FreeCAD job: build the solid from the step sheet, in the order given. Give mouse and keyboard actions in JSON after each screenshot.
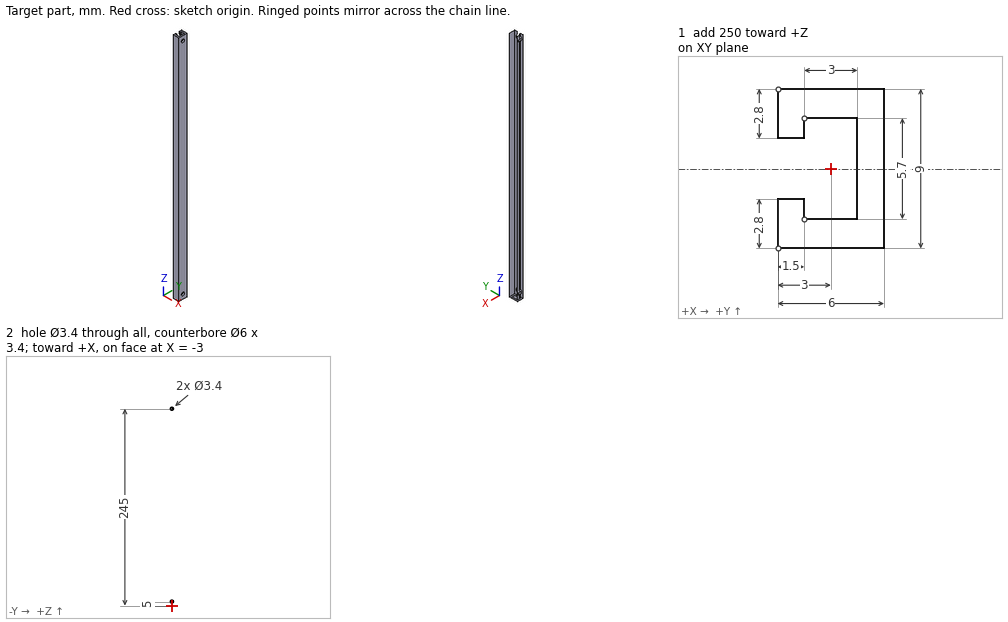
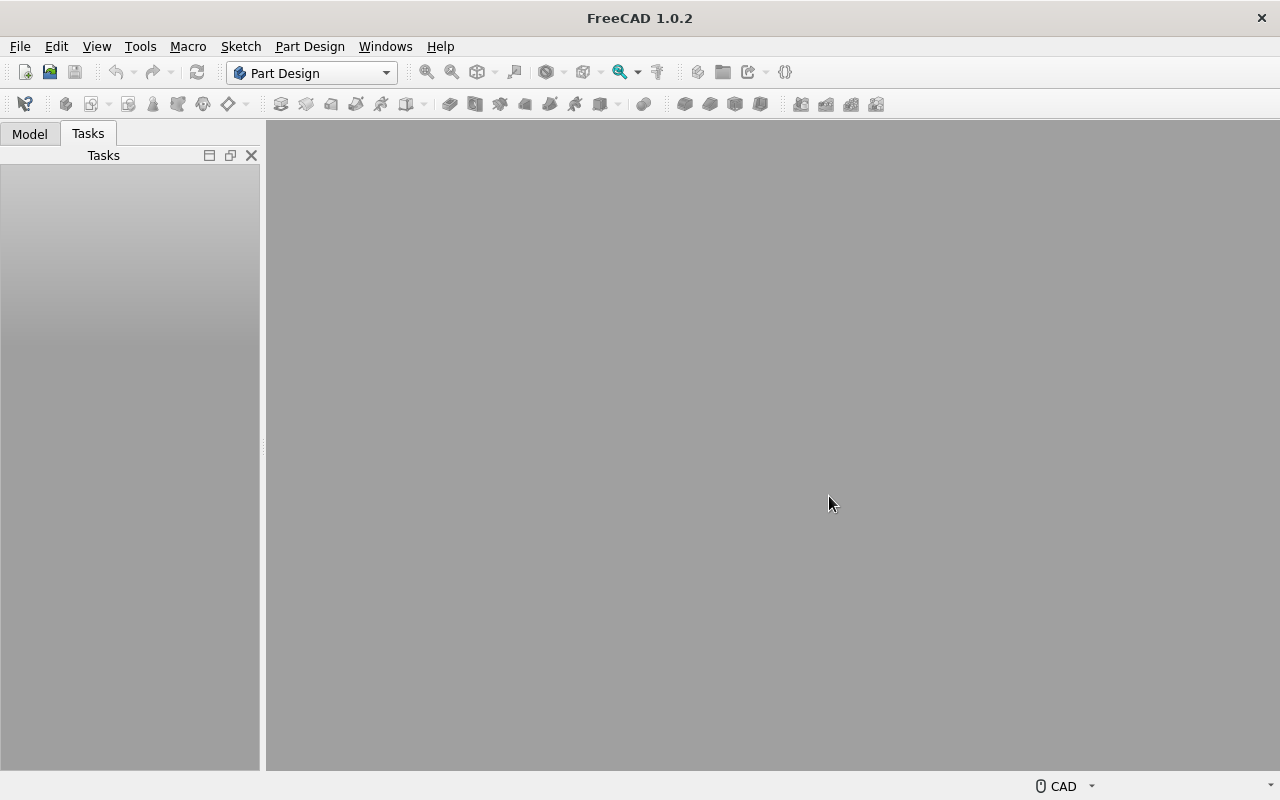
{"action": "left_click", "coordinate": [25, 72]}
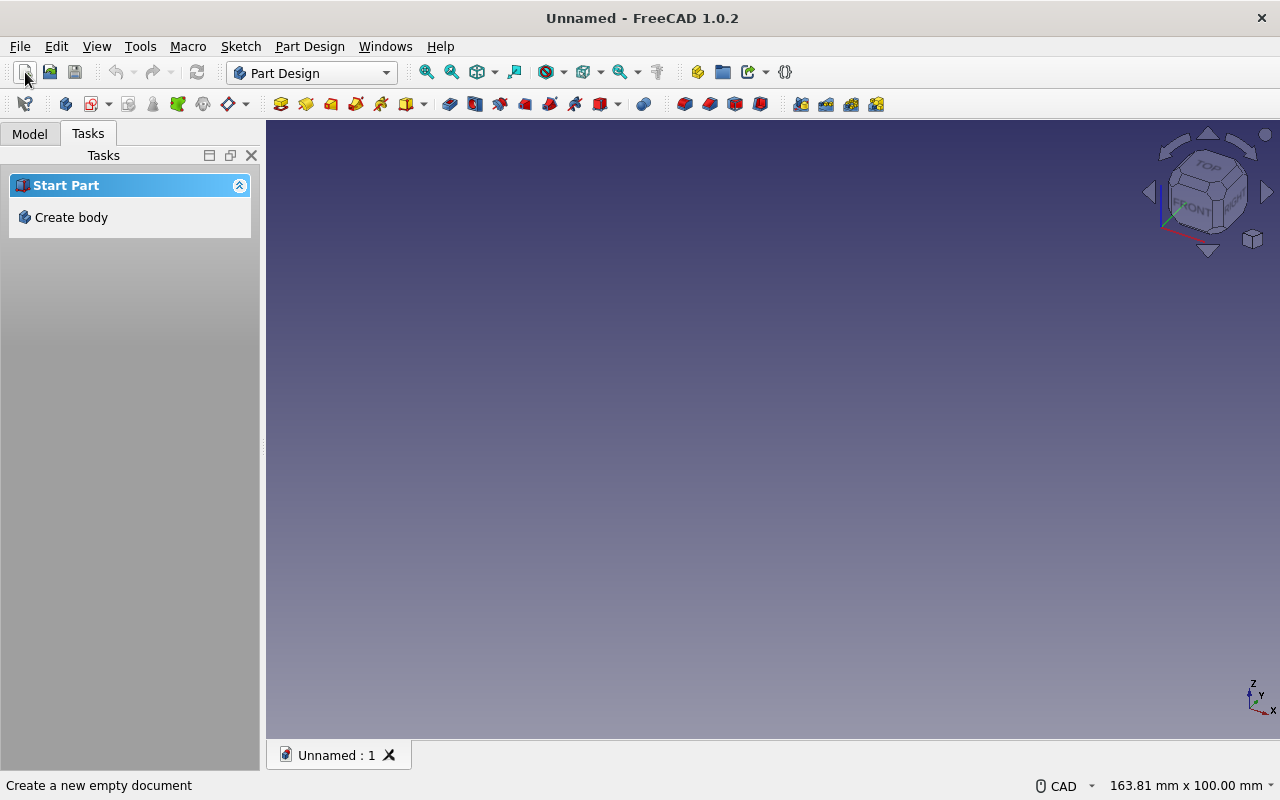
{"action": "left_click", "coordinate": [90, 104]}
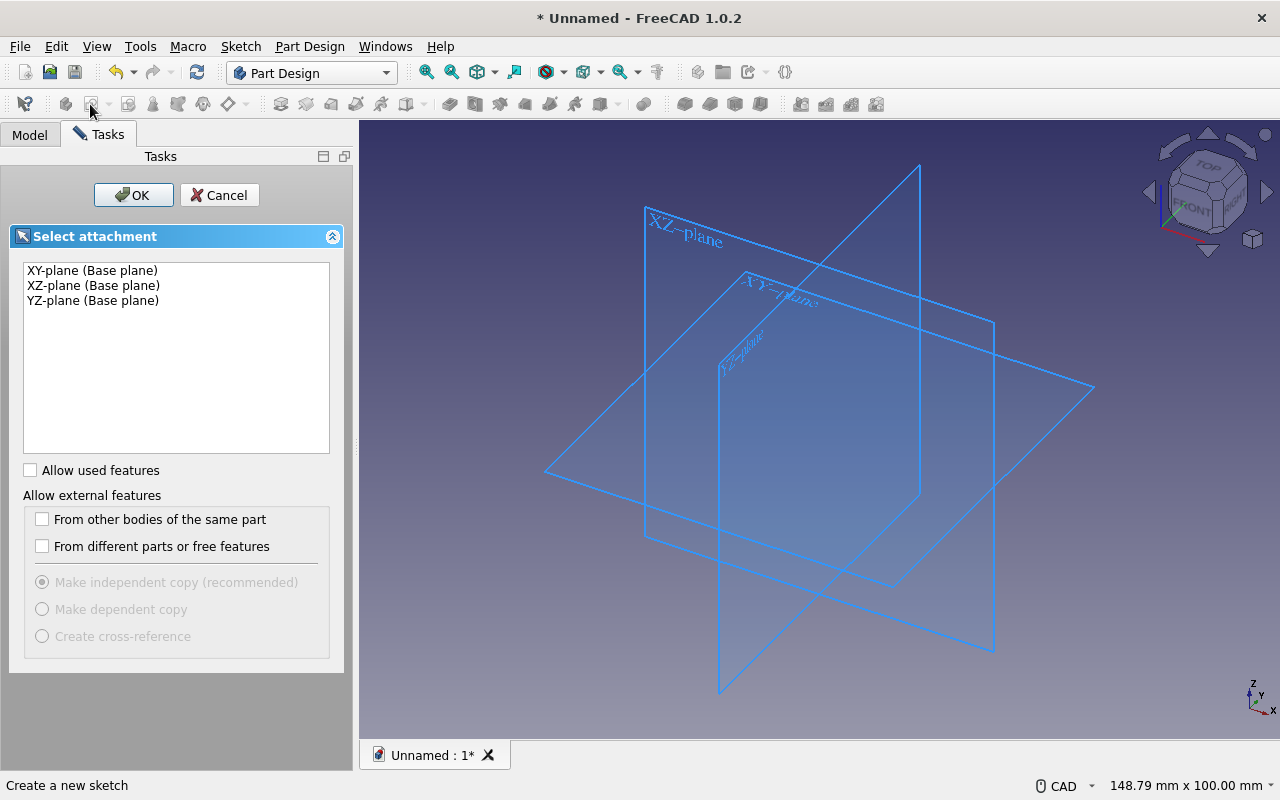
{"action": "left_click", "coordinate": [84, 270]}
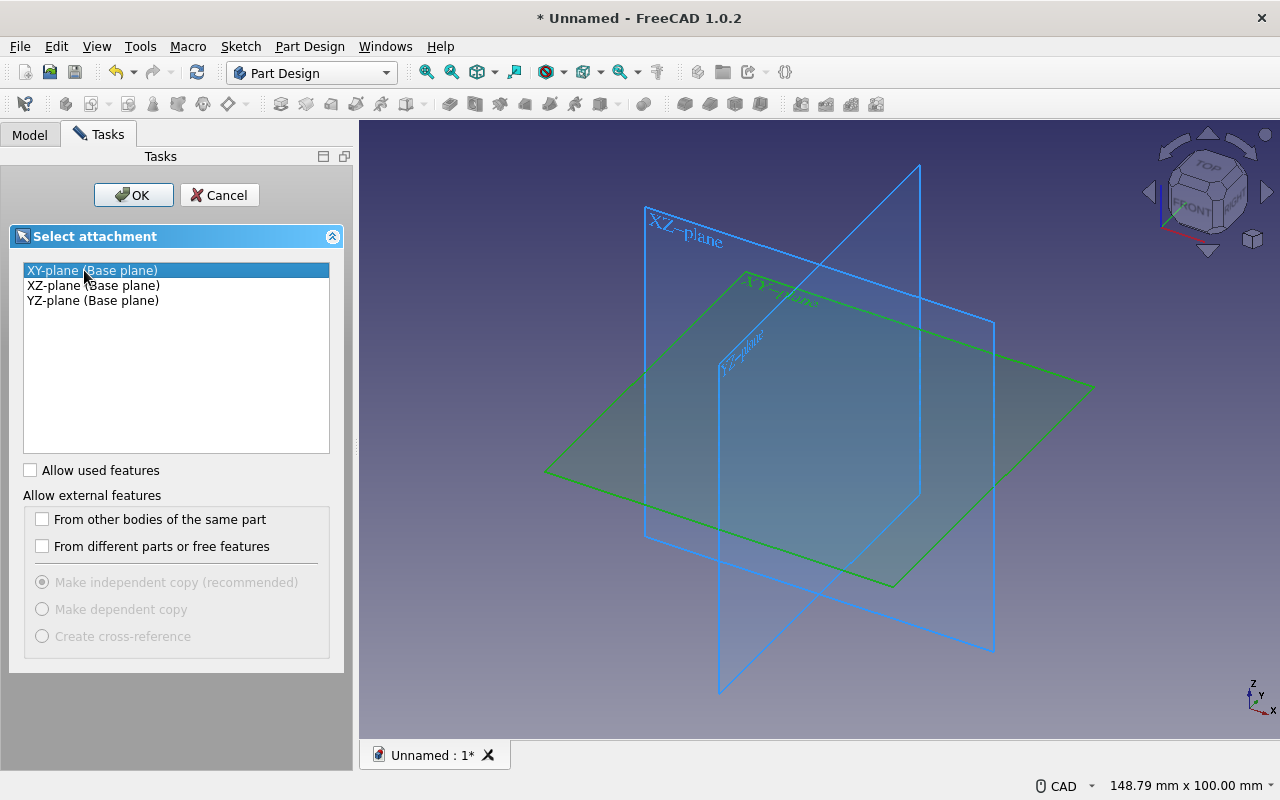
{"action": "left_click", "coordinate": [134, 195]}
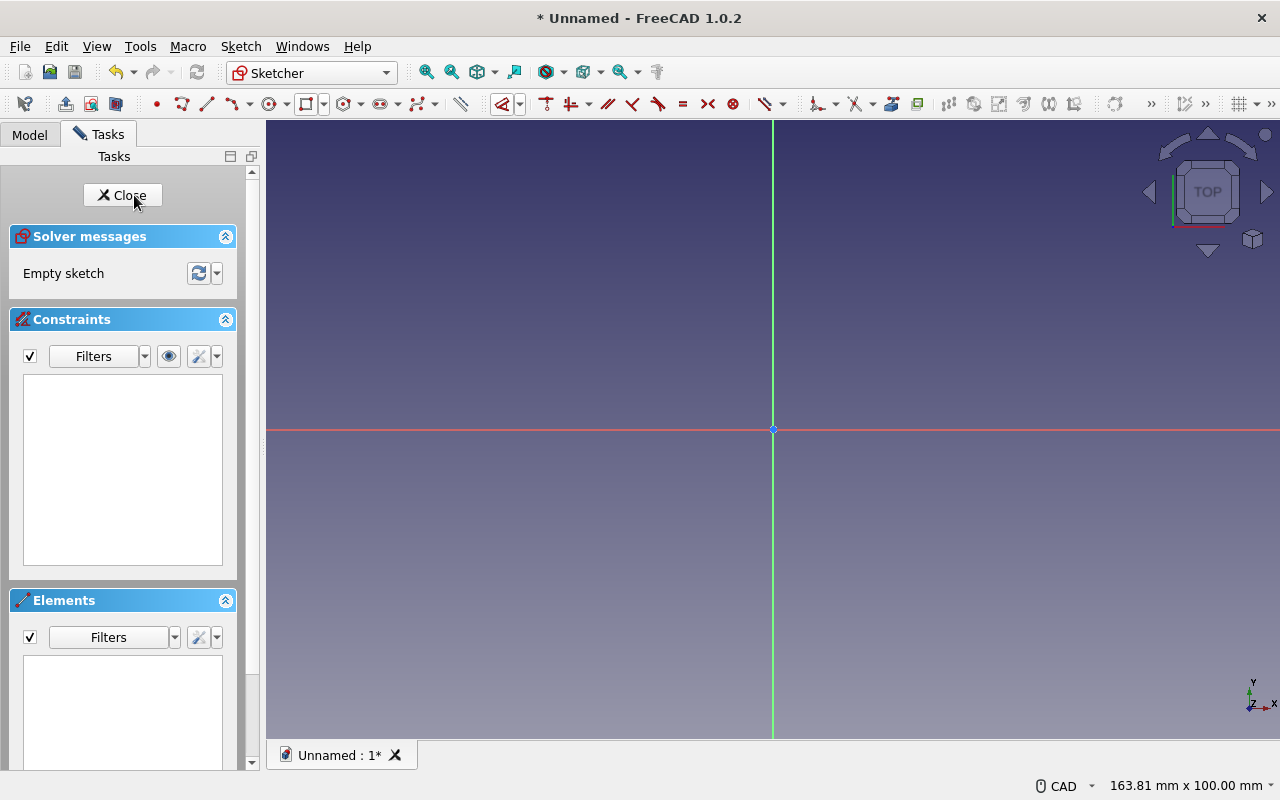
{"action": "scroll", "coordinate": [784, 430], "scroll_direction": "up", "scroll_amount": 10}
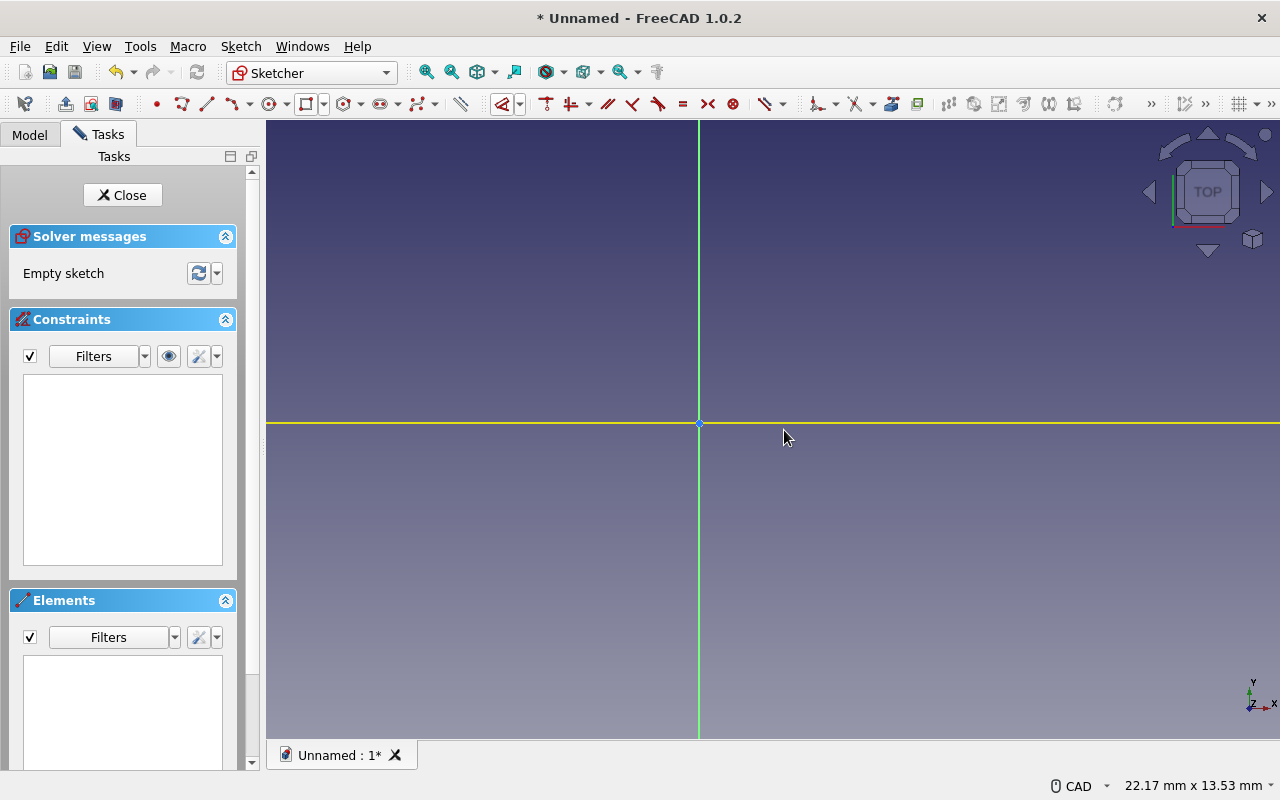
{"action": "key", "text": "g m"}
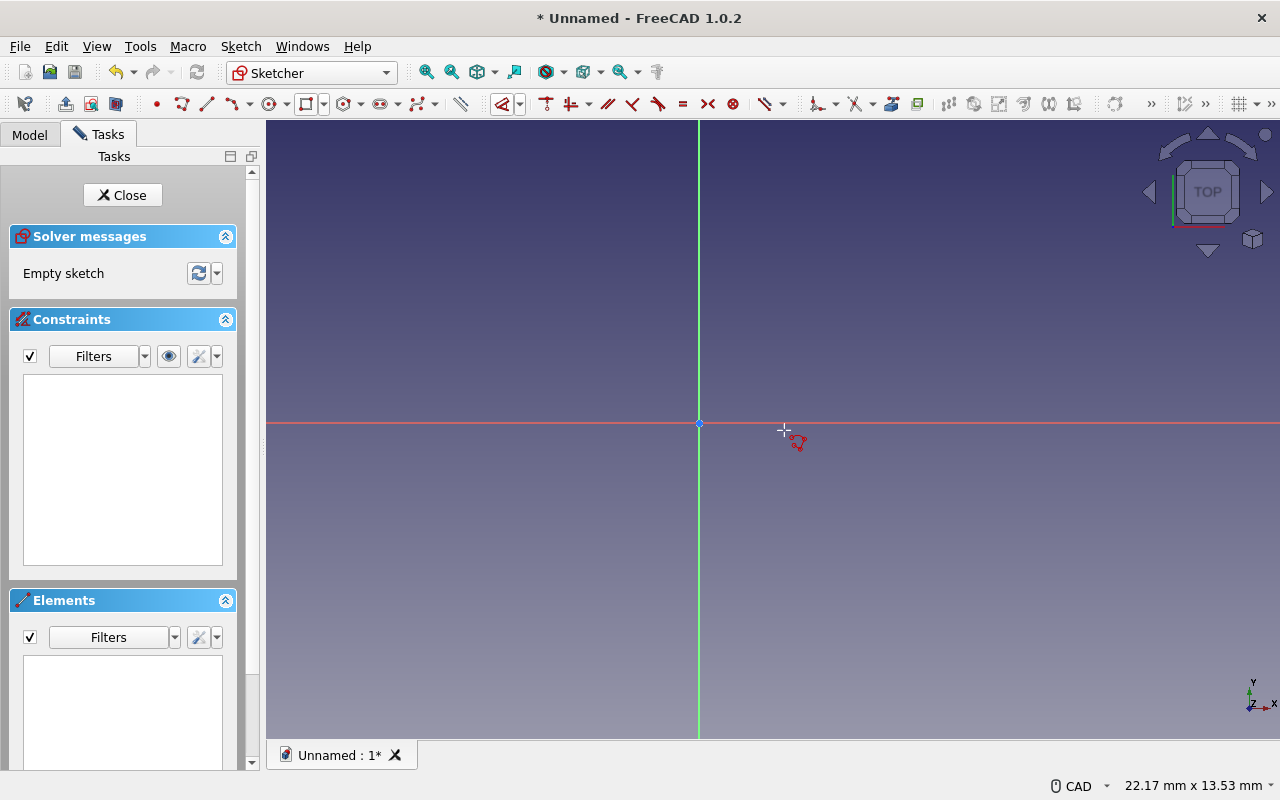
{"action": "left_click", "coordinate": [631, 345]}
{"action": "left_click", "coordinate": [631, 293]}
{"action": "left_click", "coordinate": [768, 293]}
{"action": "left_click", "coordinate": [768, 553]}
{"action": "left_click", "coordinate": [631, 553]}
{"action": "left_click", "coordinate": [631, 501]}
{"action": "left_click", "coordinate": [562, 501]}
{"action": "left_click", "coordinate": [562, 629]}
{"action": "left_click", "coordinate": [837, 629]}
{"action": "left_click", "coordinate": [837, 217]}
{"action": "left_click", "coordinate": [562, 217]}
{"action": "left_click", "coordinate": [562, 345]}
{"action": "left_click", "coordinate": [631, 346]}
{"action": "key", "text": "Escape"}
{"action": "key", "text": "Escape"}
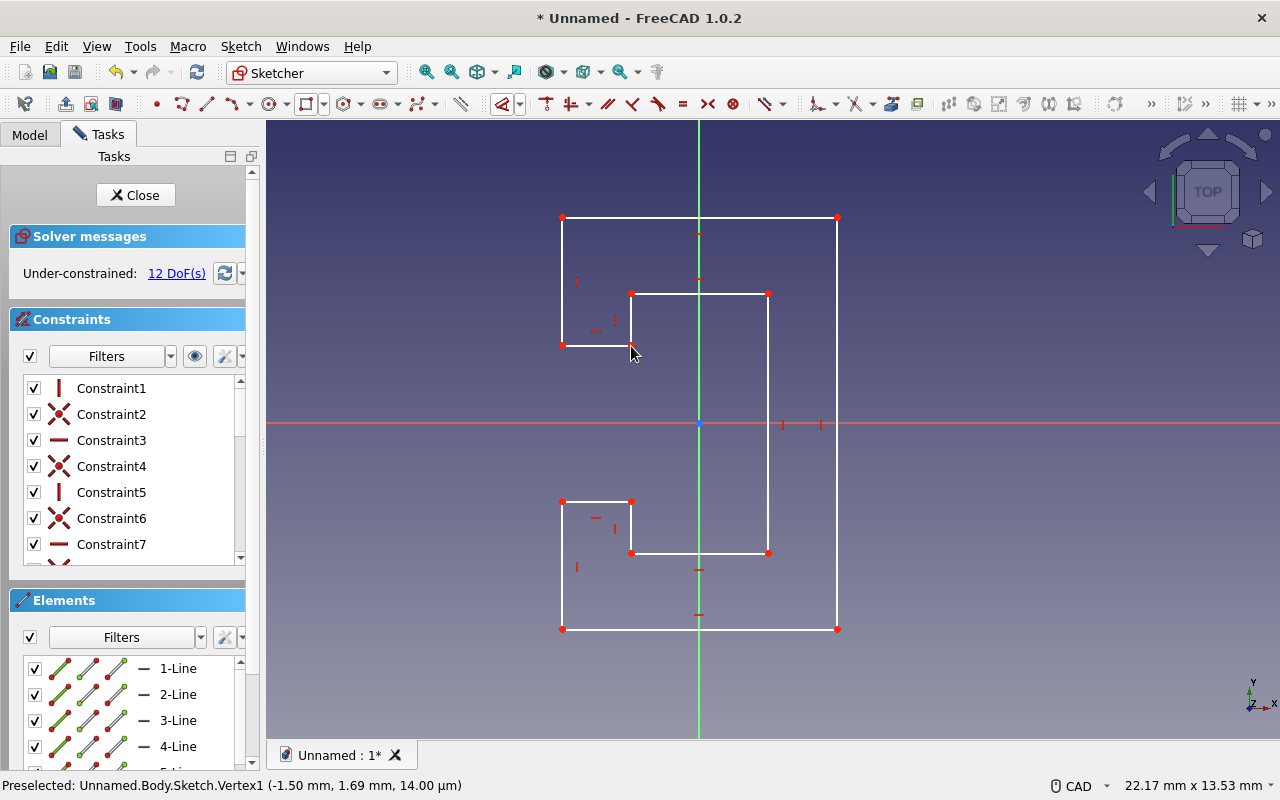
{"action": "left_click", "coordinate": [631, 294]}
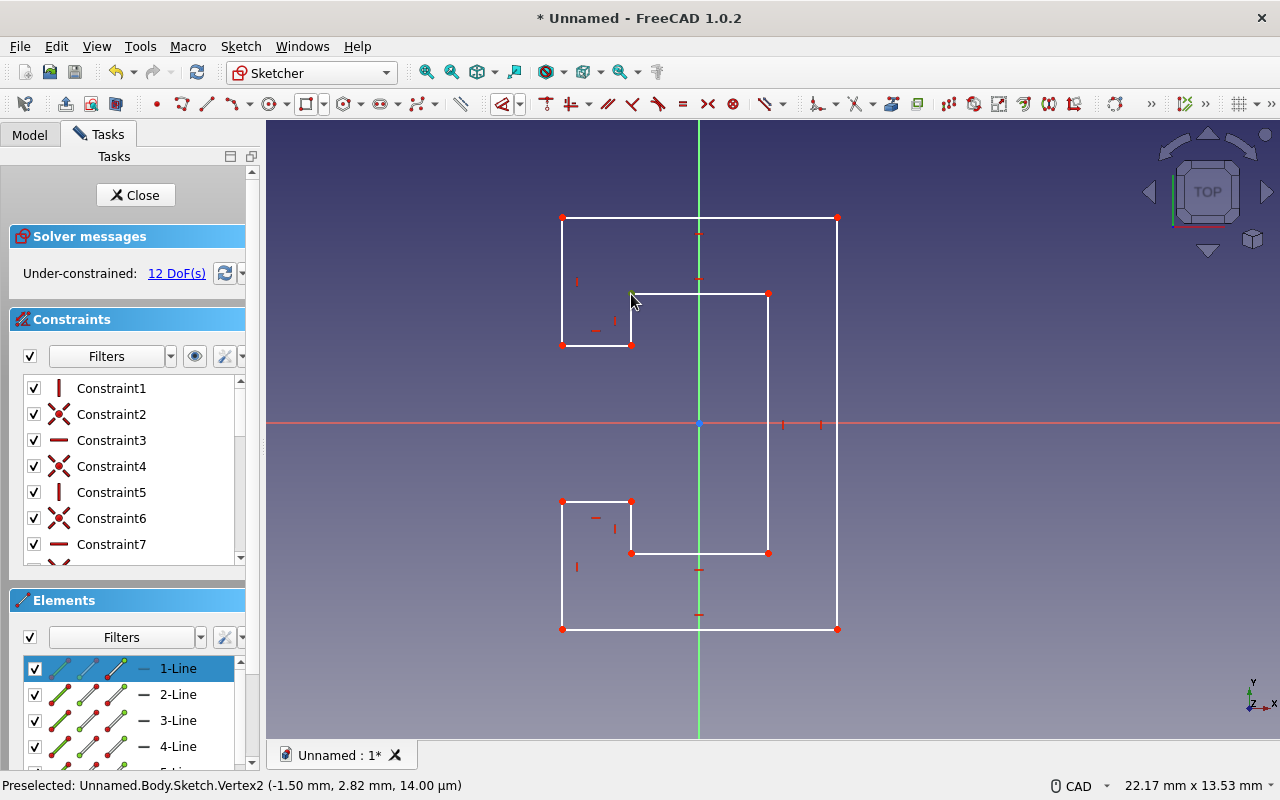
{"action": "left_click", "coordinate": [631, 554]}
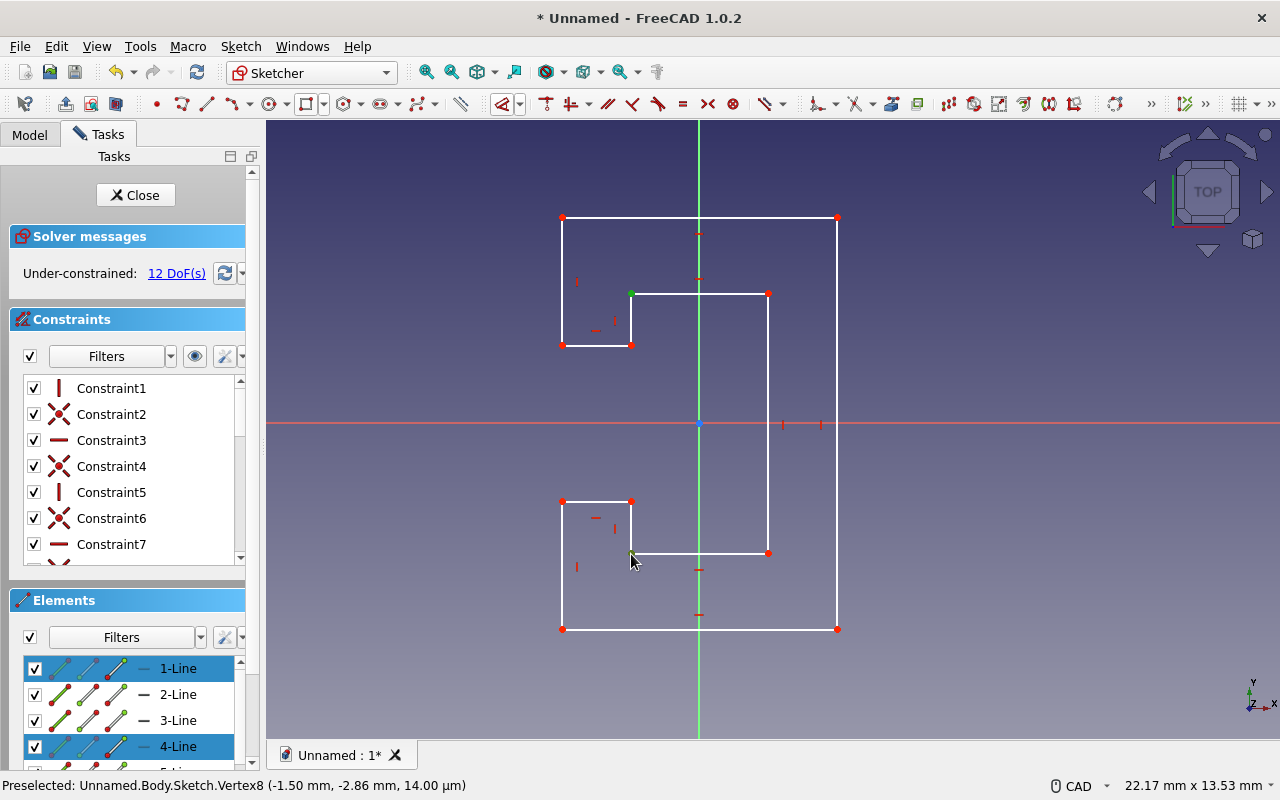
{"action": "left_click", "coordinate": [353, 423]}